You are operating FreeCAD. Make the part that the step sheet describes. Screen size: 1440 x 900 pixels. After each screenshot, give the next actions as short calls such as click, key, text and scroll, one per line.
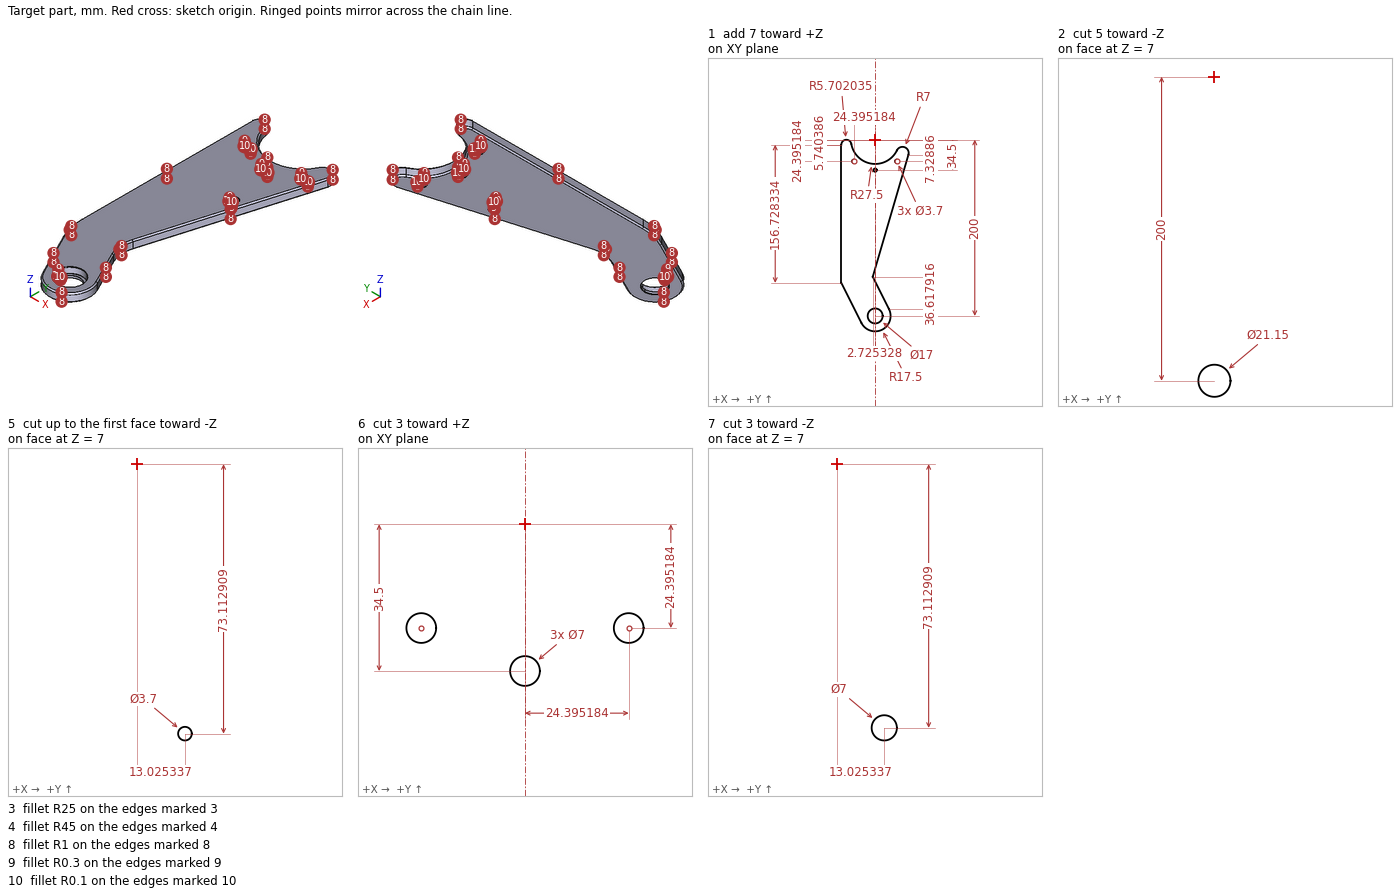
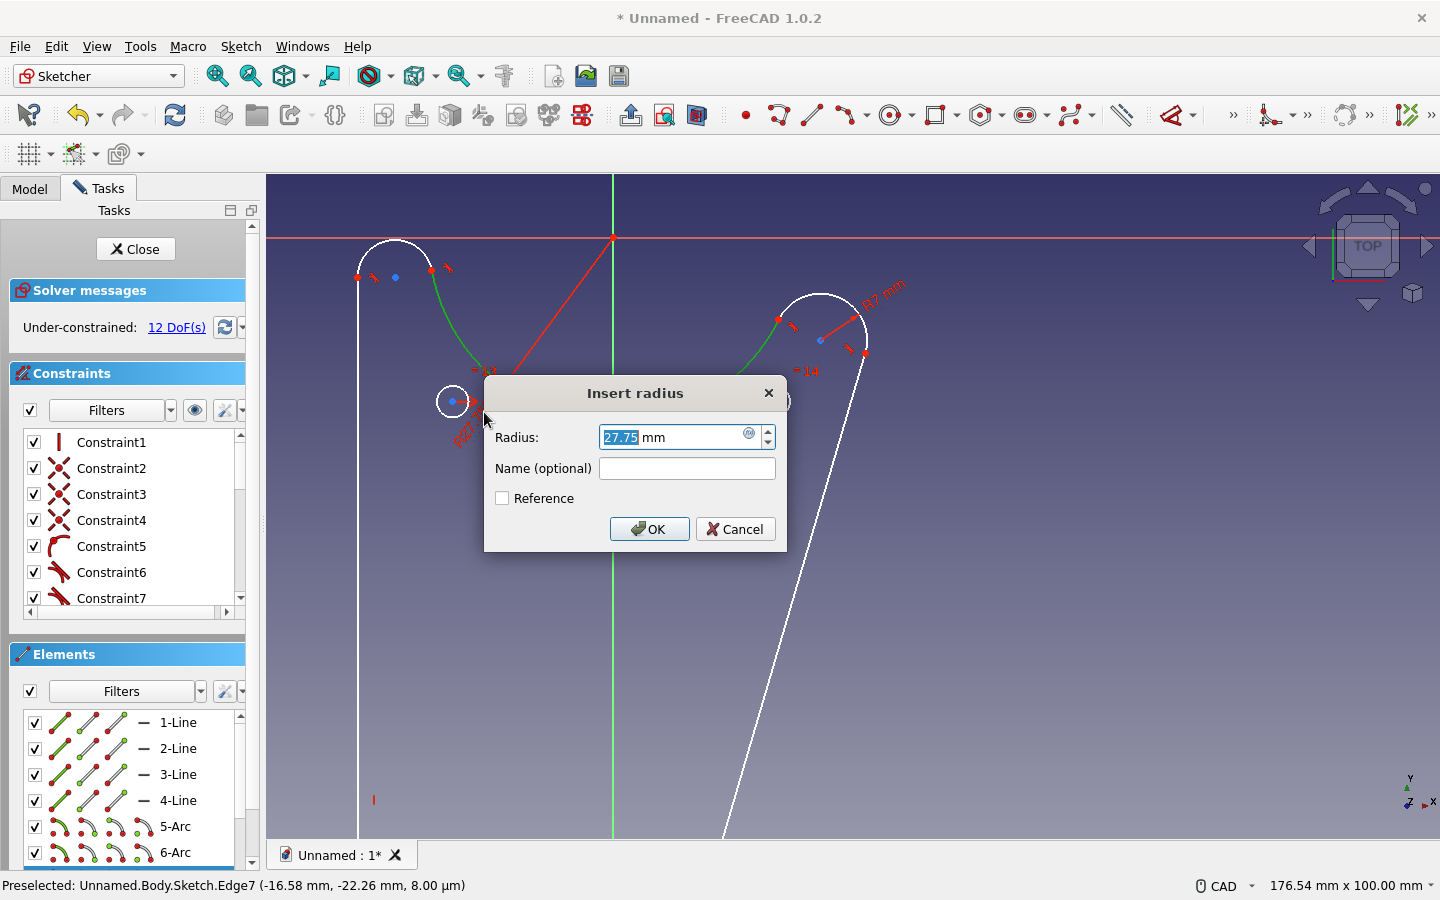
text(27.5)
key(Return)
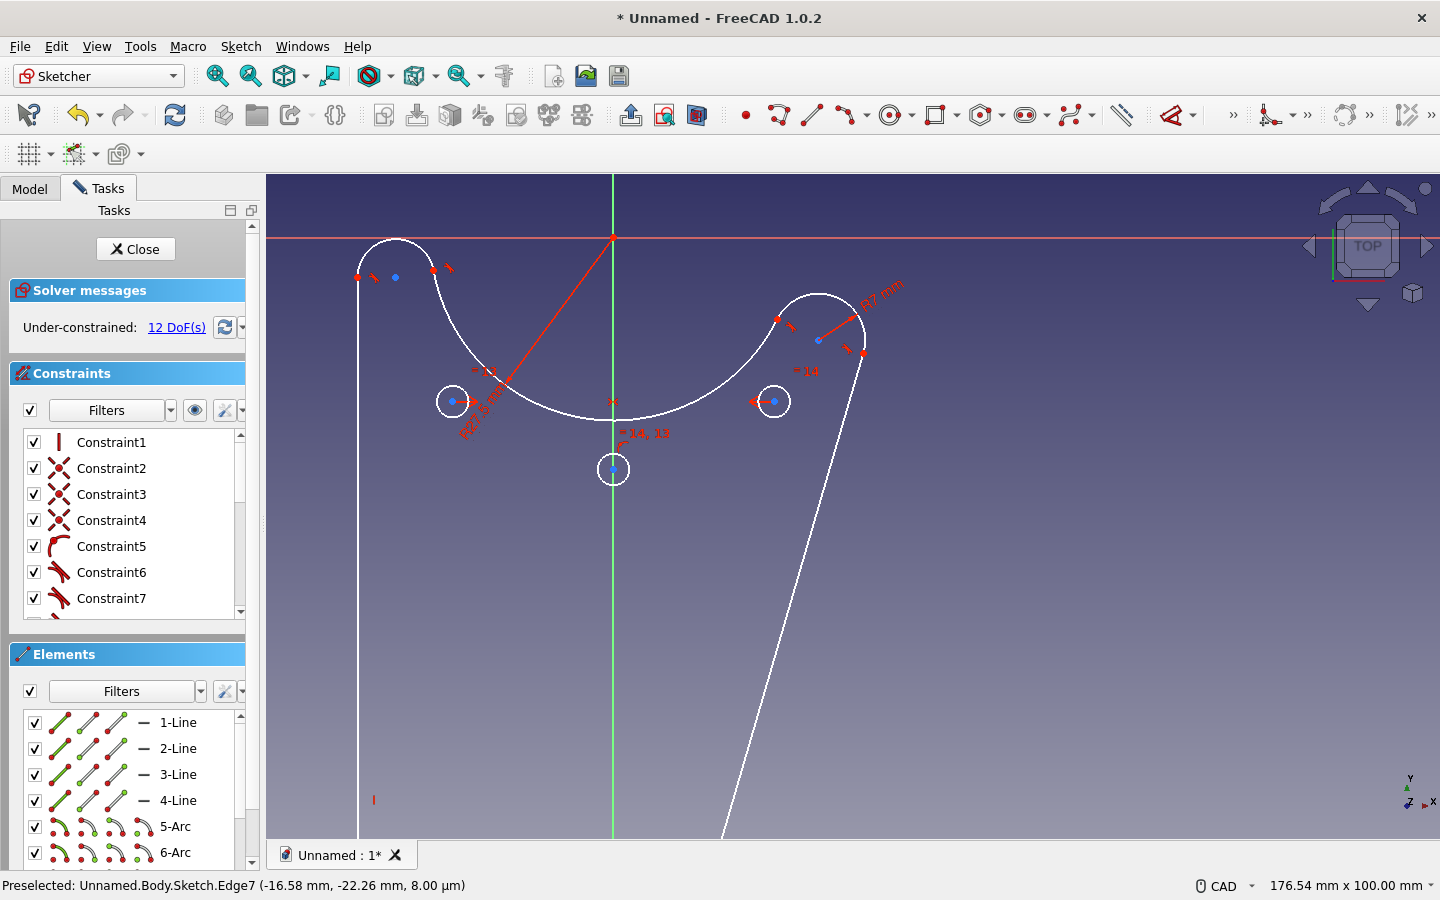
scroll(372, 248, up, 2)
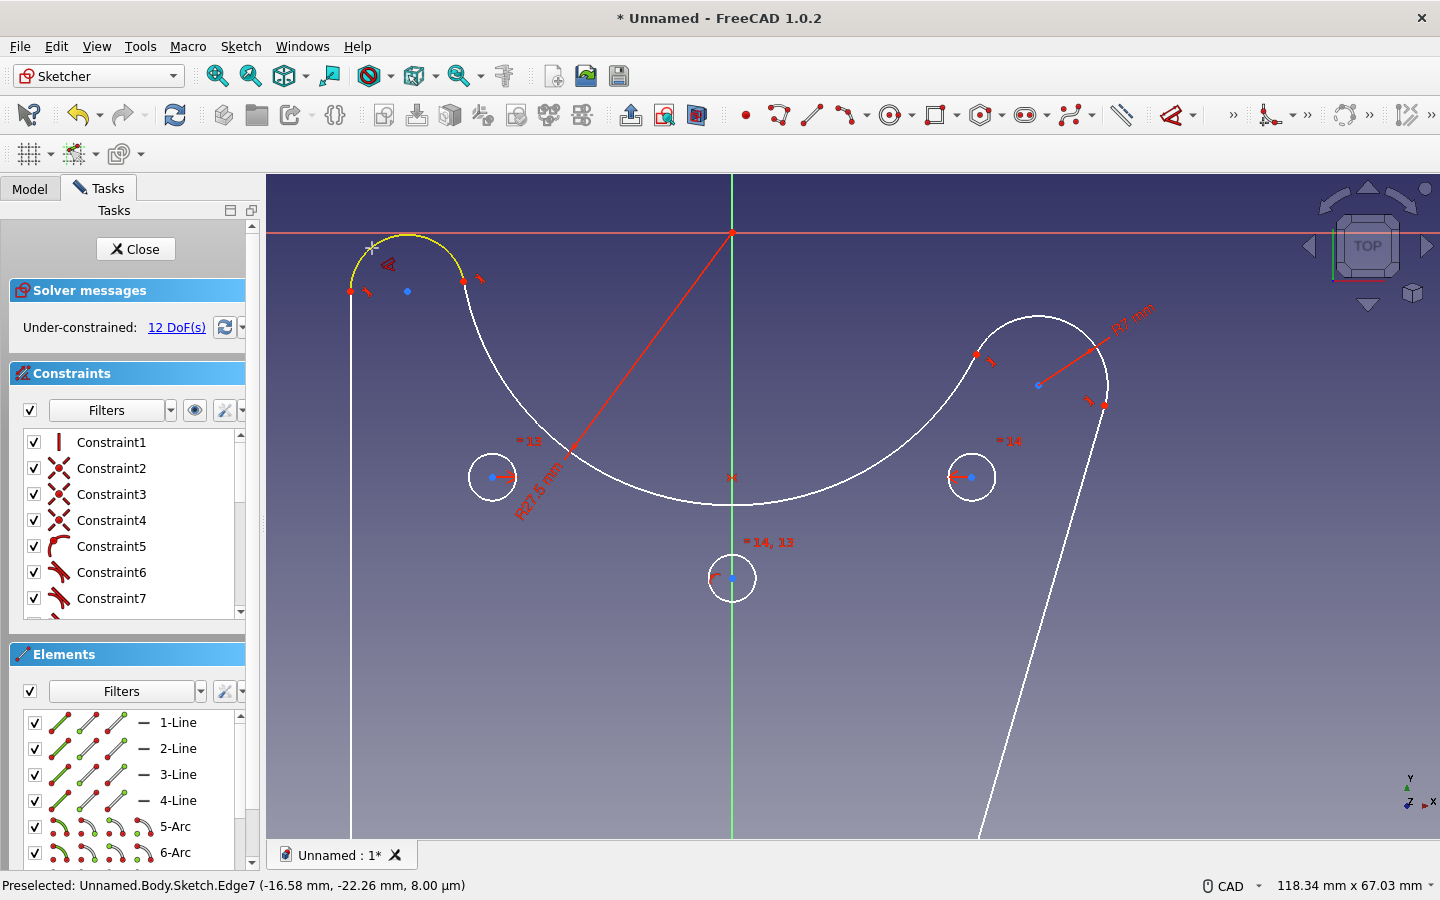
click(372, 248)
click(392, 205)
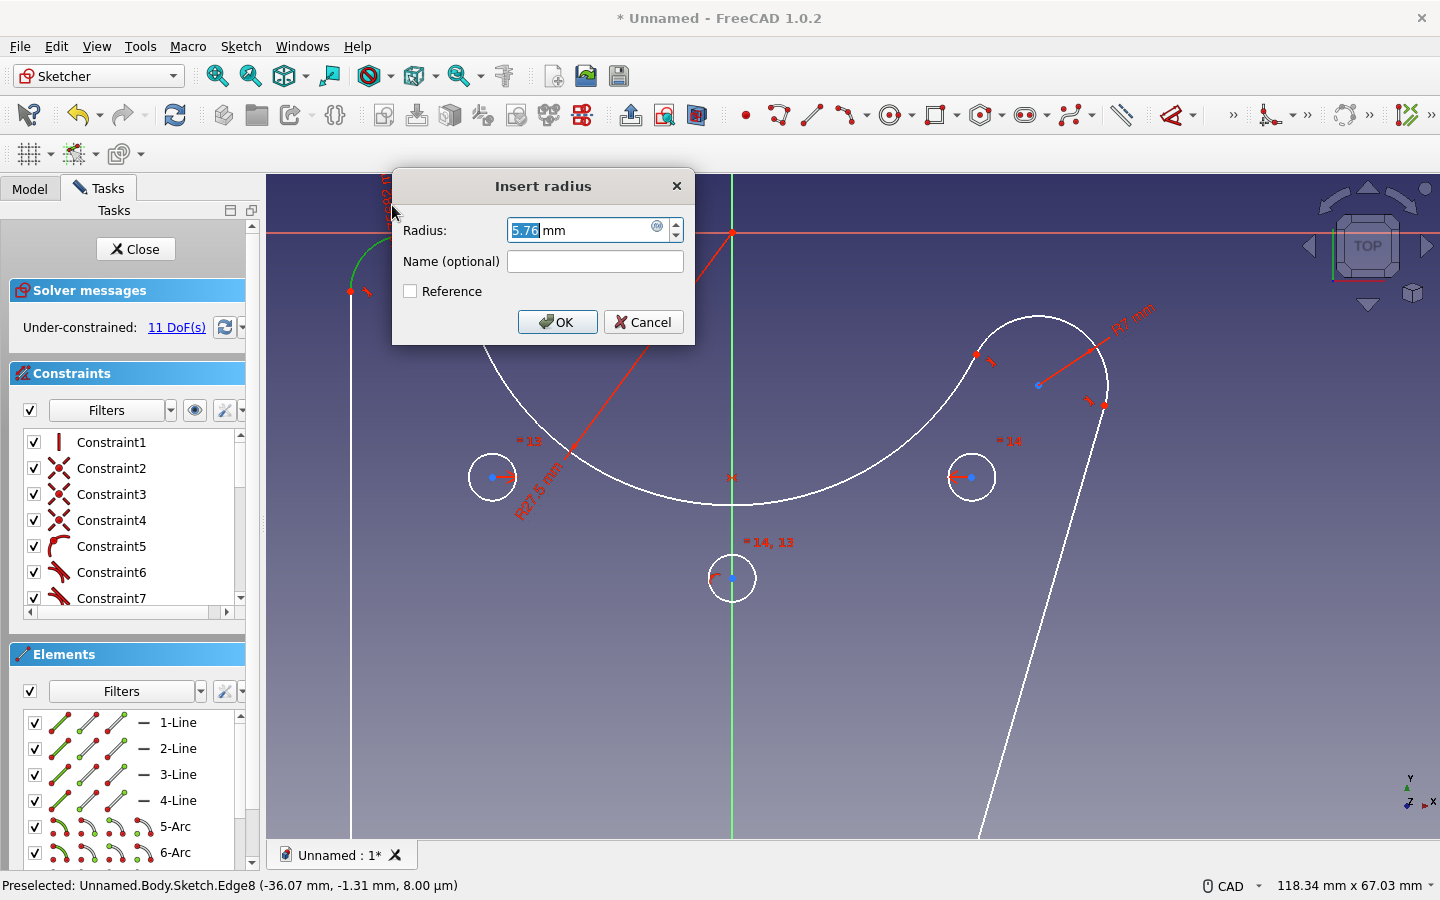
text(5.702035)
key(Return)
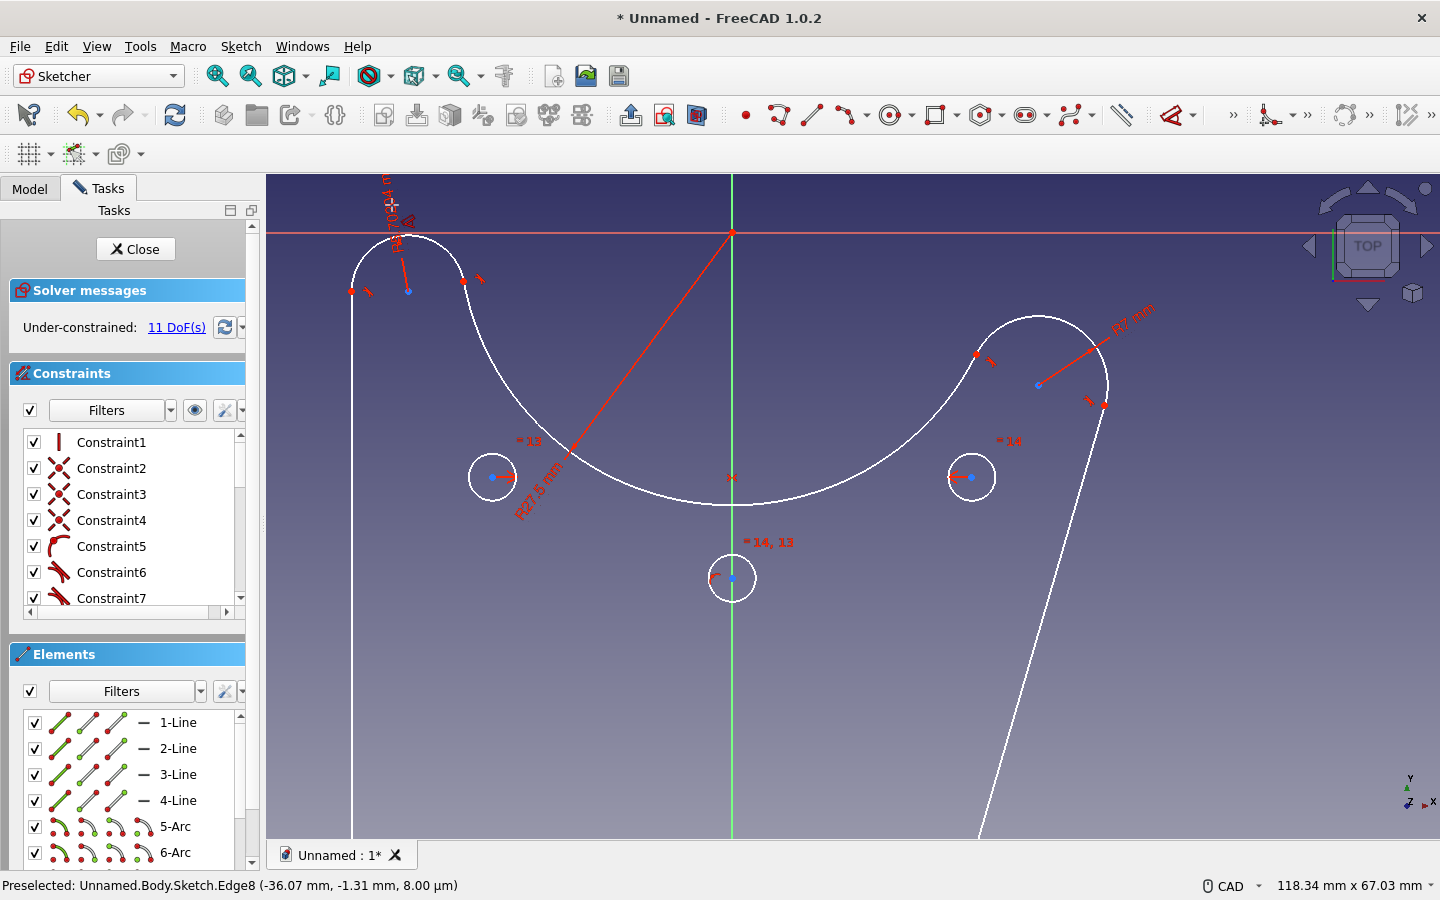
scroll(799, 305, down, 8)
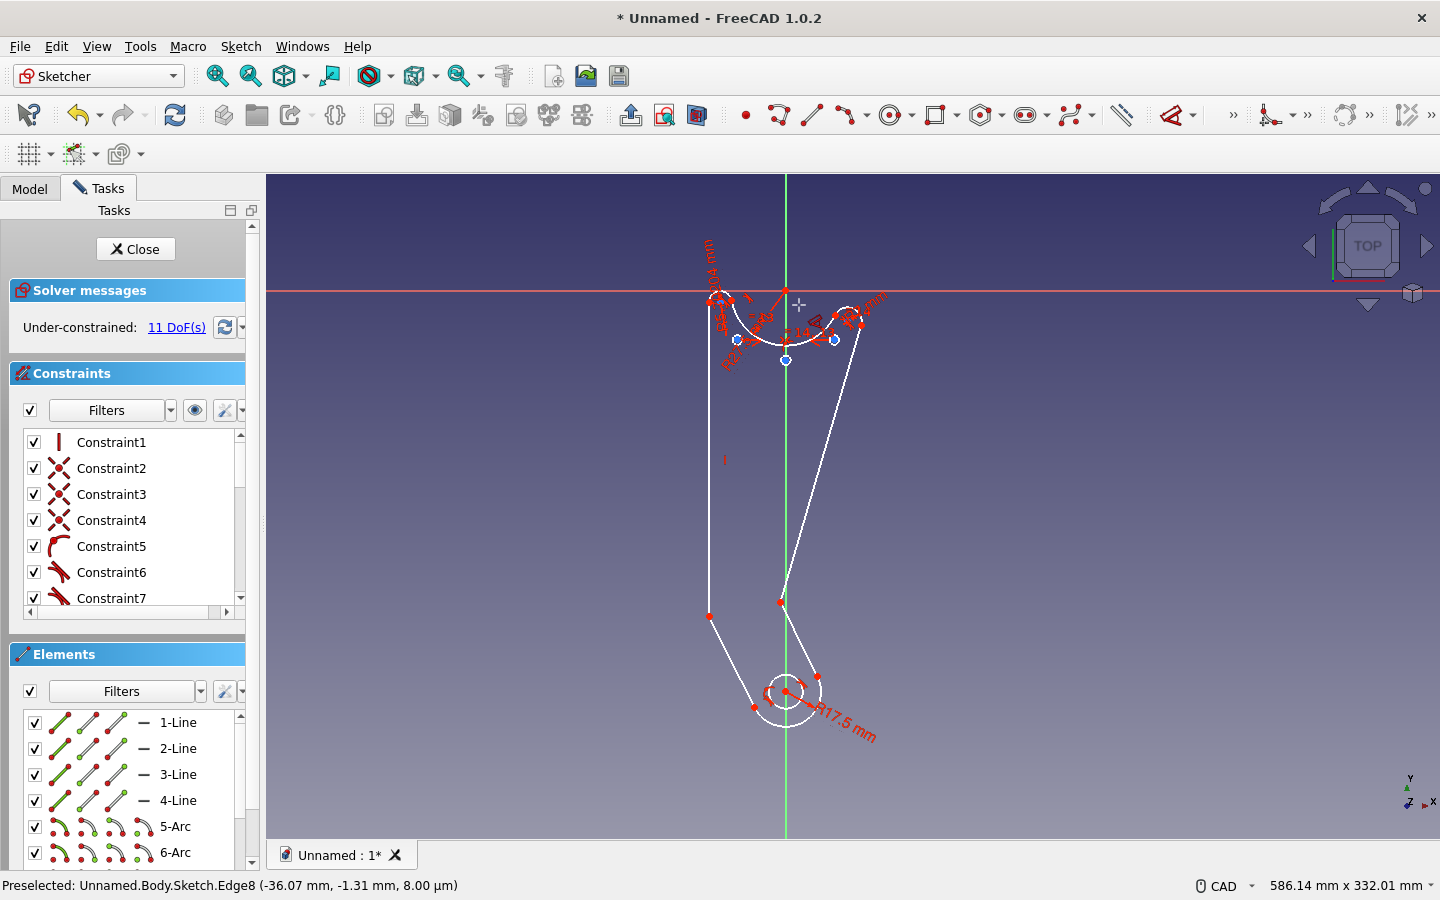
click(798, 680)
click(833, 679)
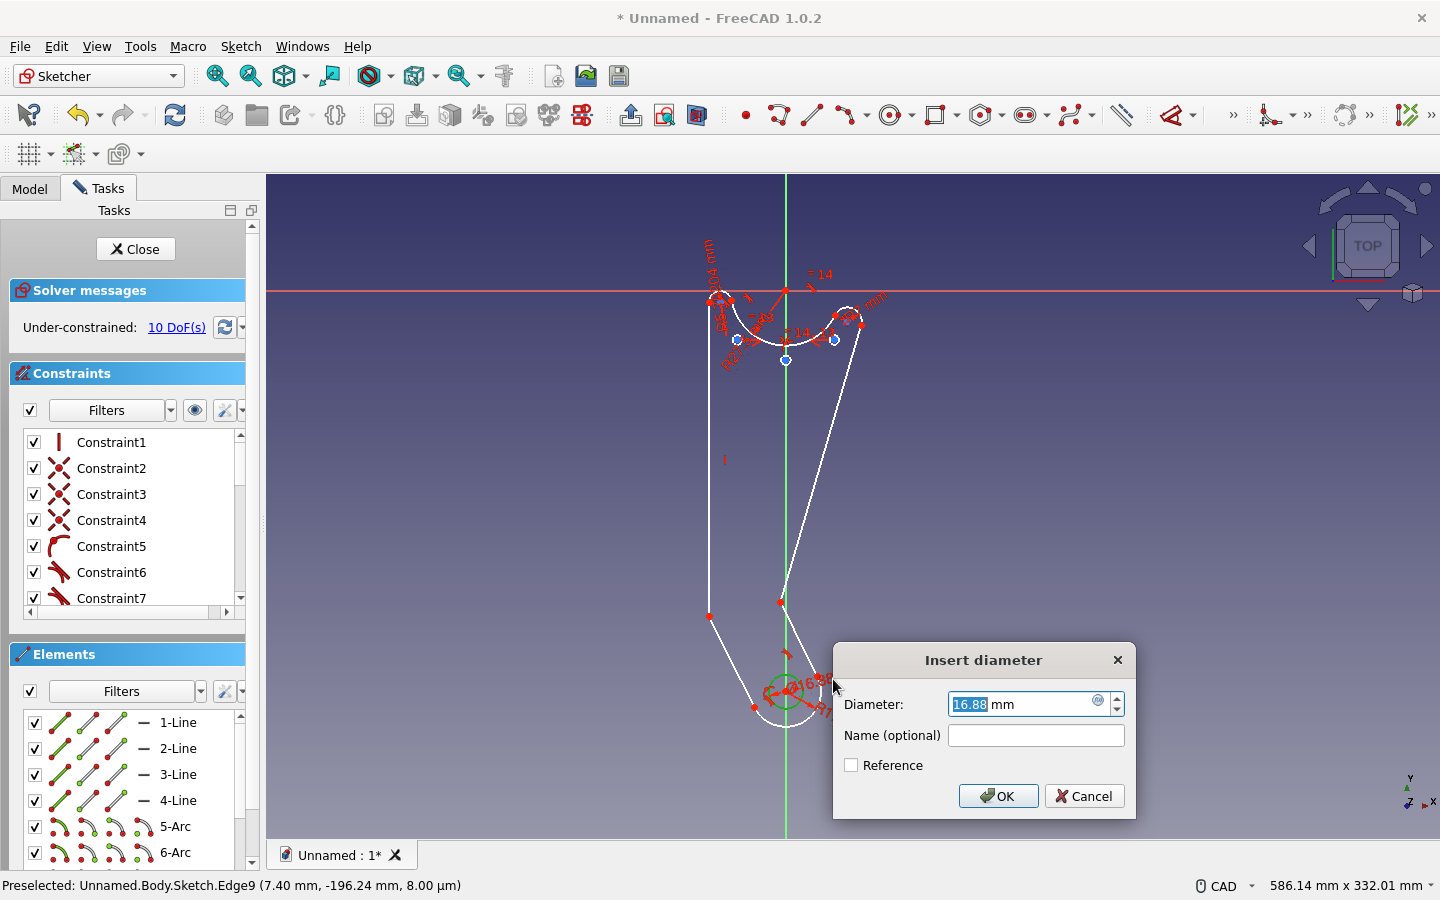
text(17)
key(Return)